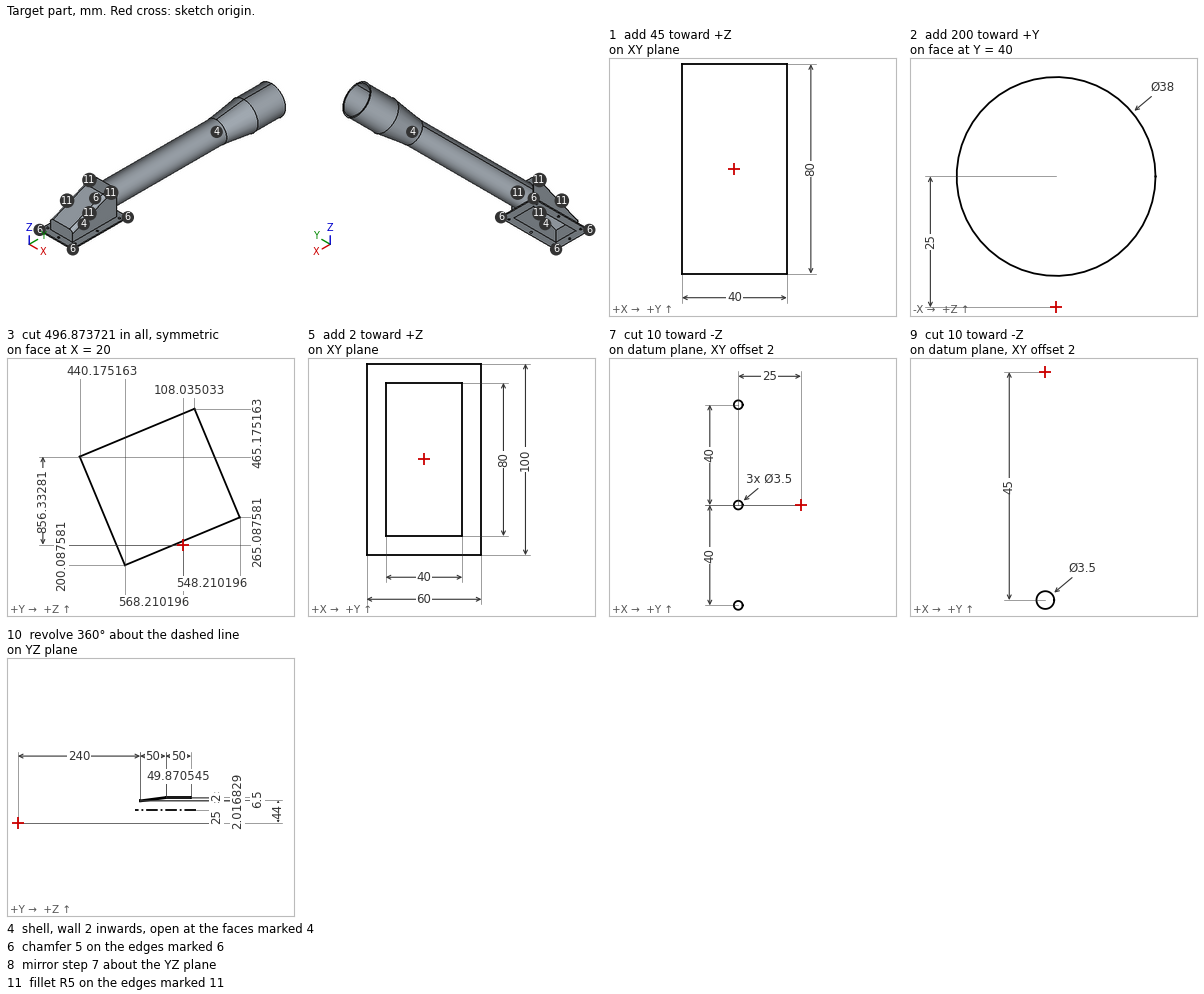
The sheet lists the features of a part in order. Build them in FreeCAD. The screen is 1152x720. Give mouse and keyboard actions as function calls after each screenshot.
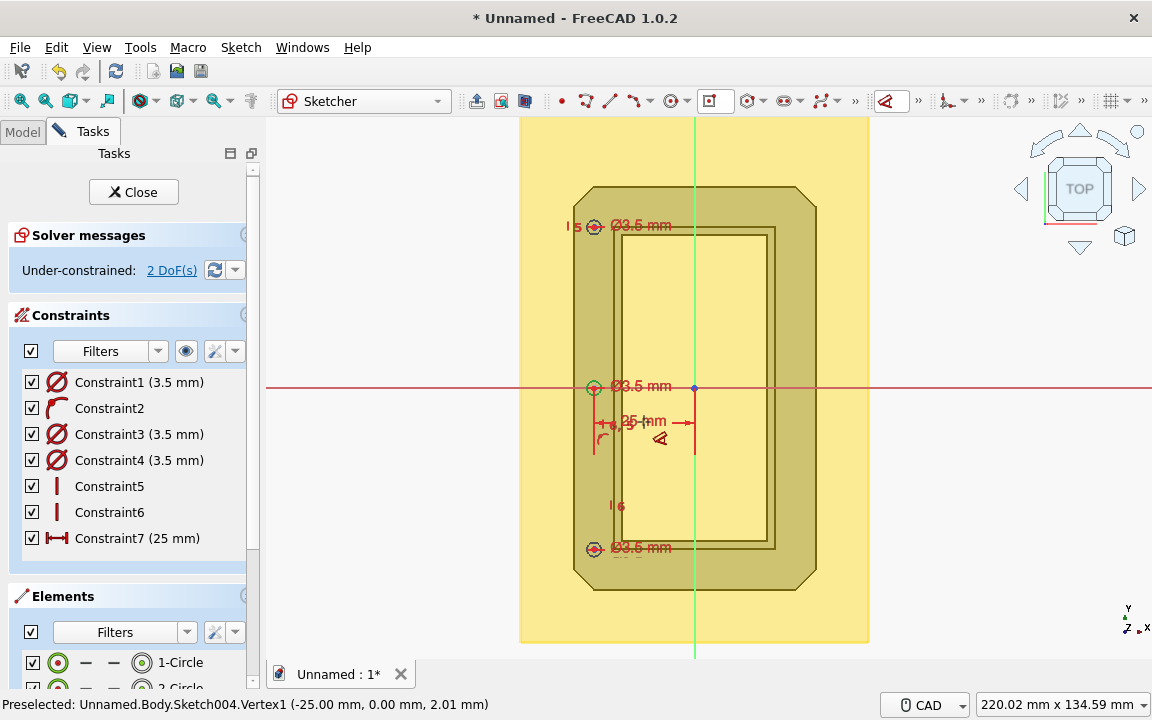
click(594, 227)
click(729, 308)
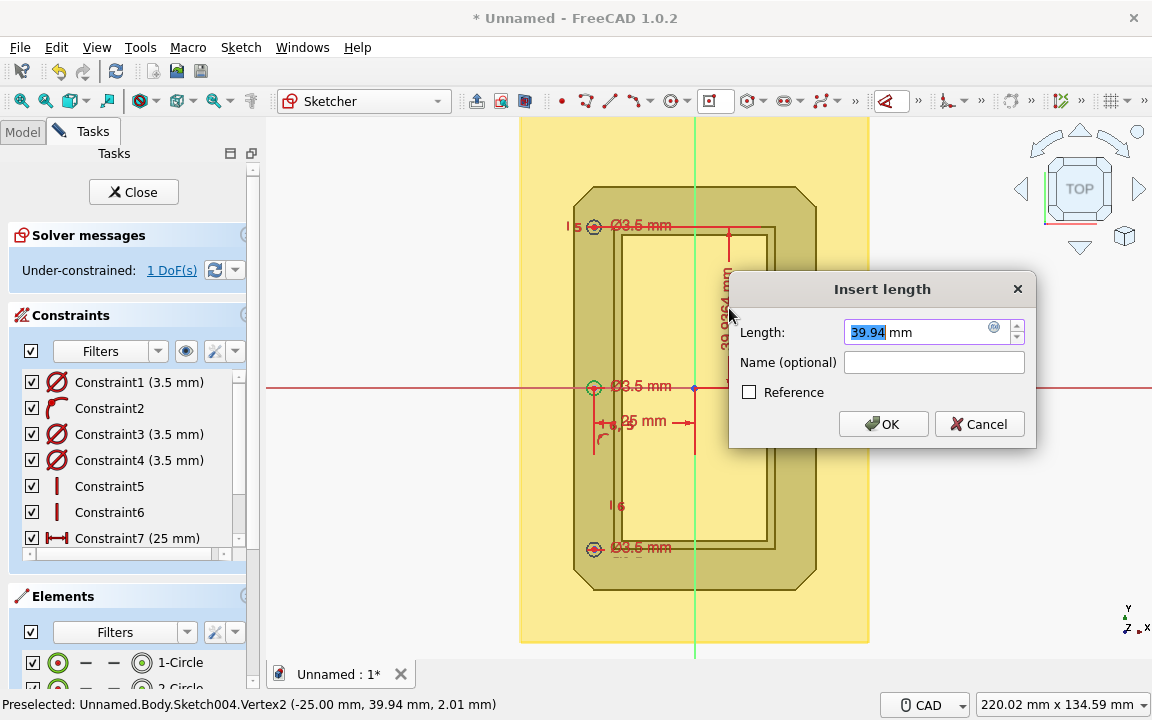
text(40)
key(Return)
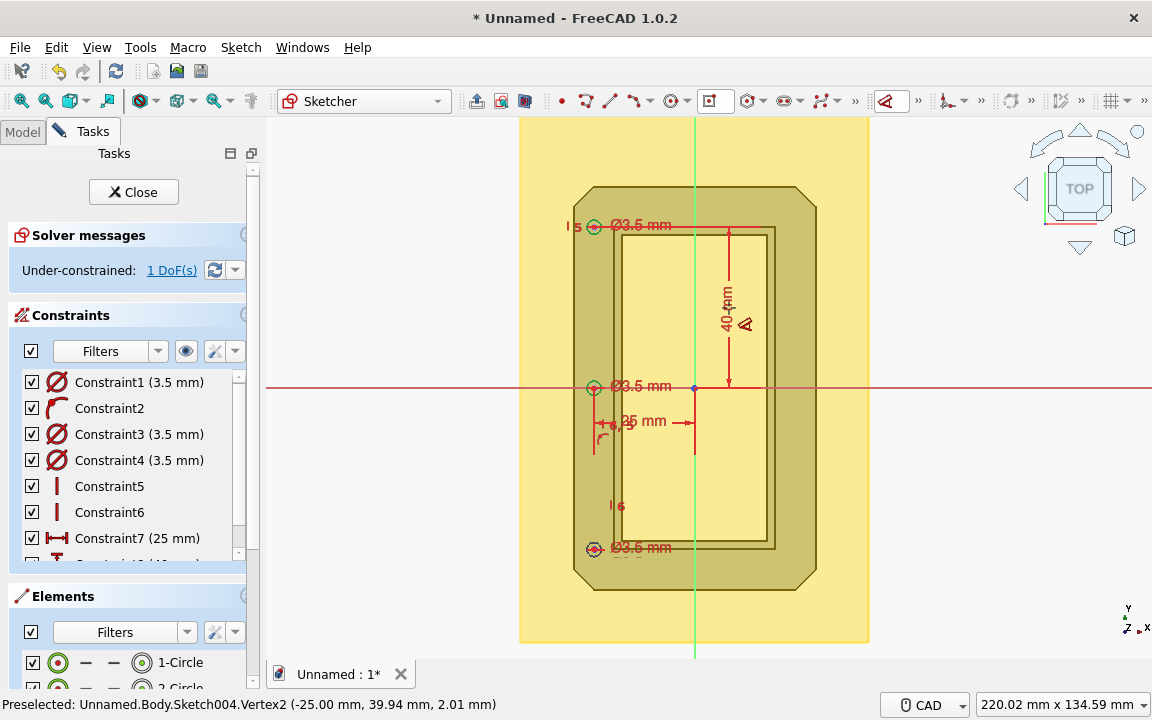
click(594, 550)
click(729, 469)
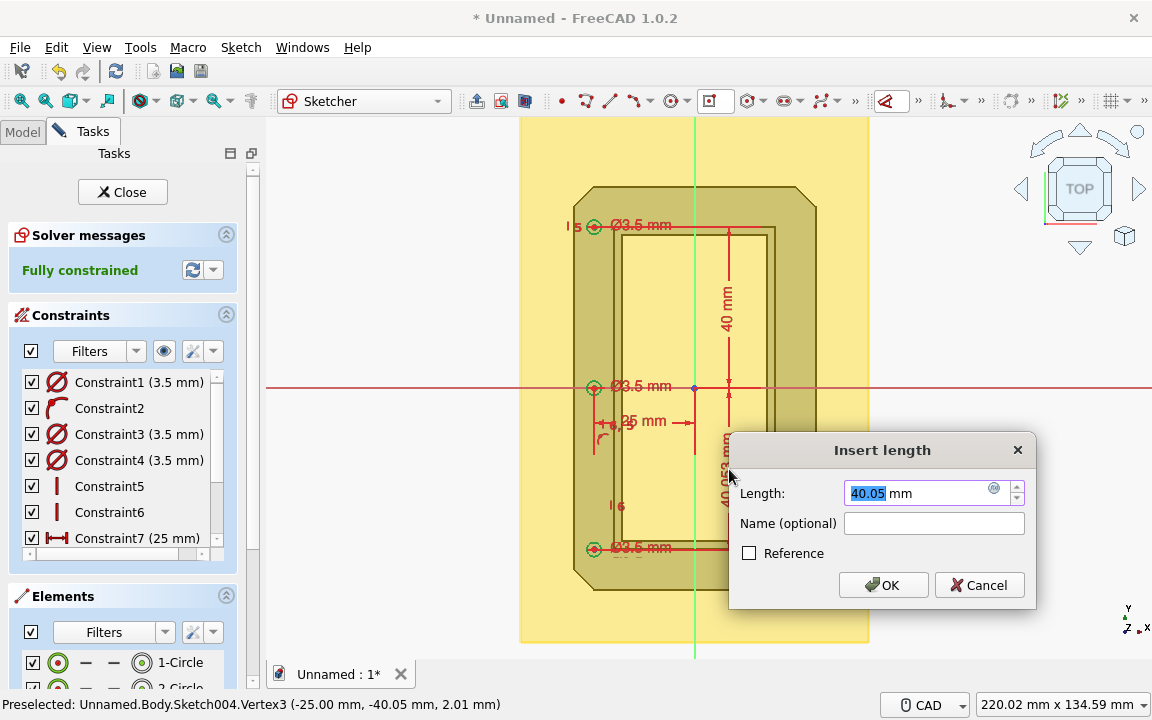
text(40)
key(Return)
key(Escape)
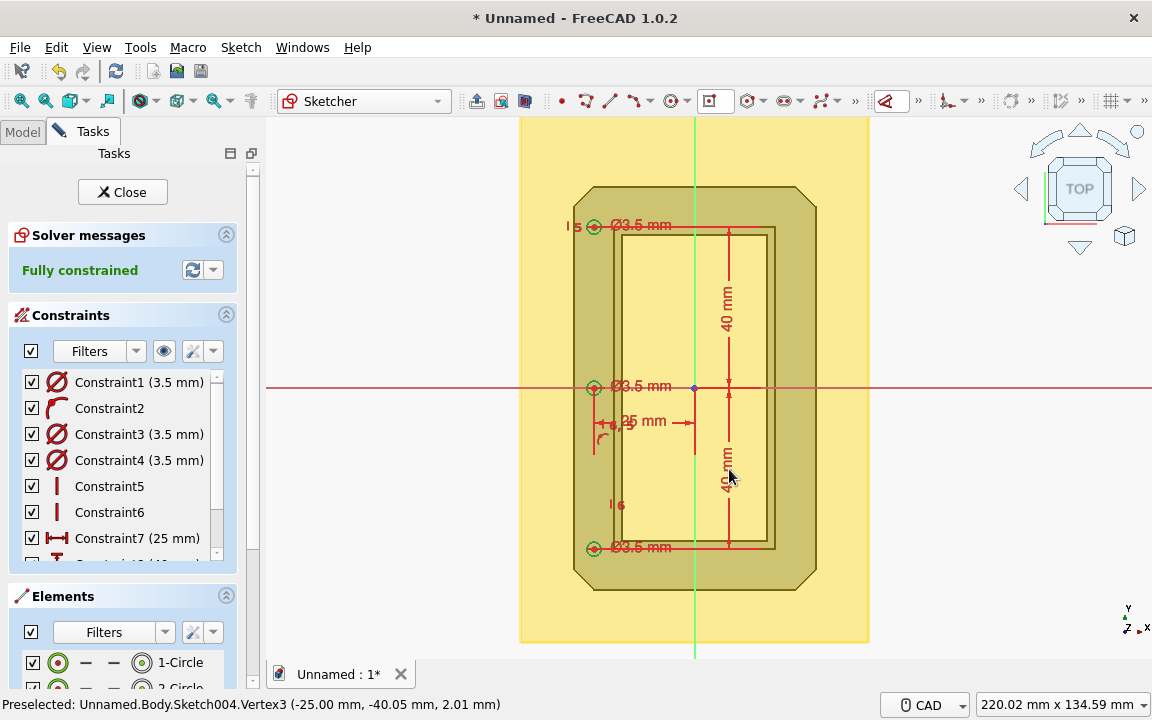
click(123, 192)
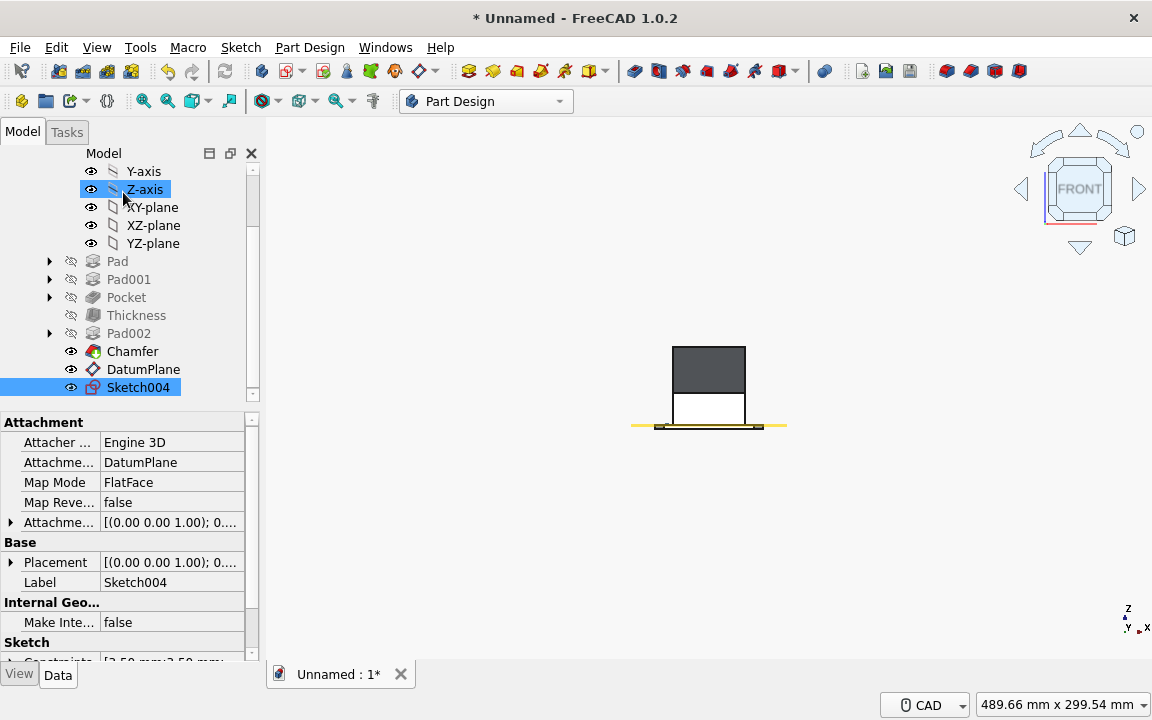
click(636, 72)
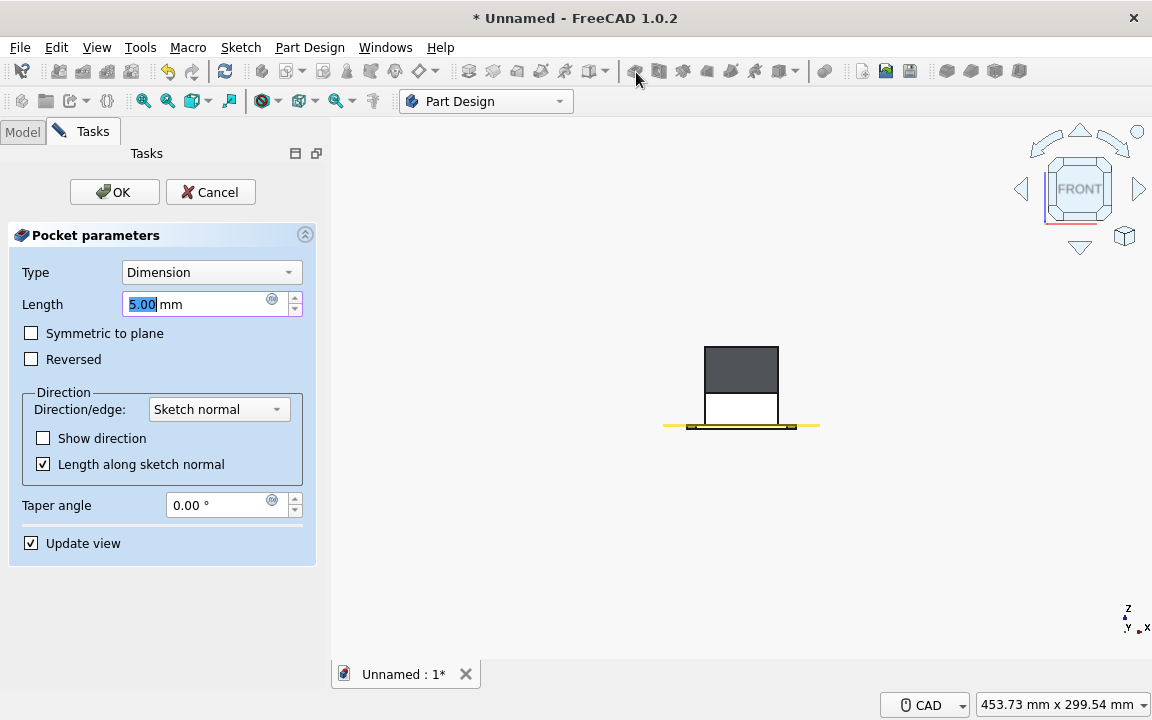
text(10)
key(Tab)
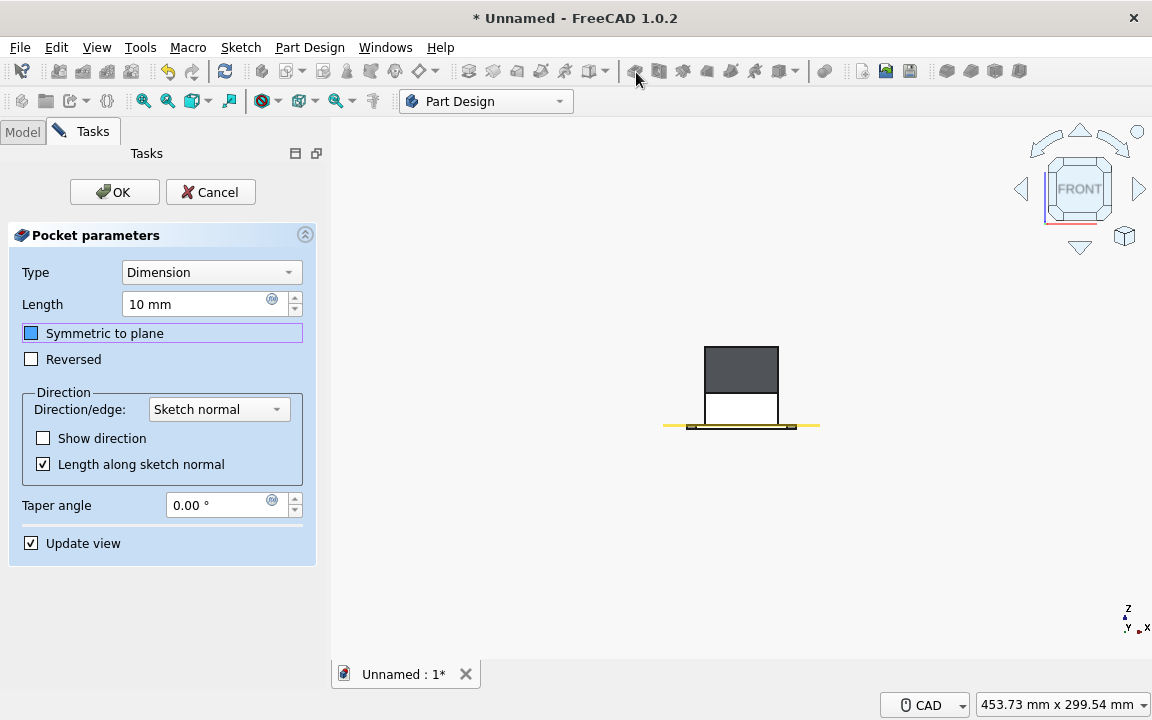
click(115, 192)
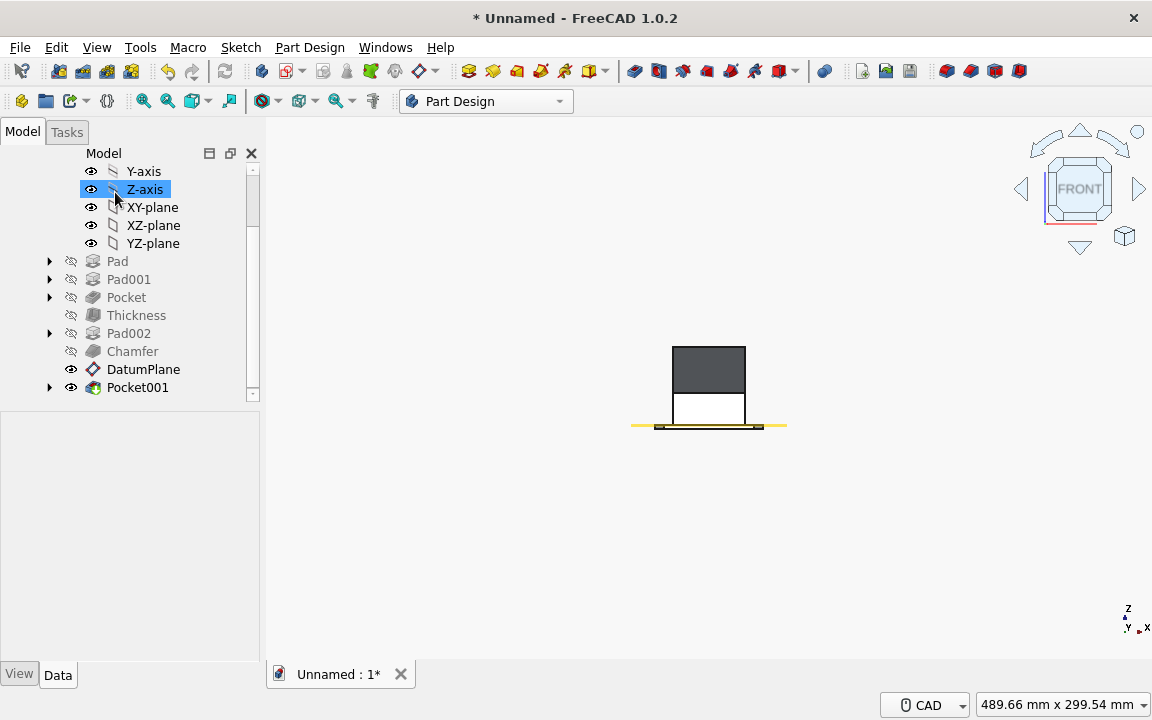
click(116, 369)
key(space)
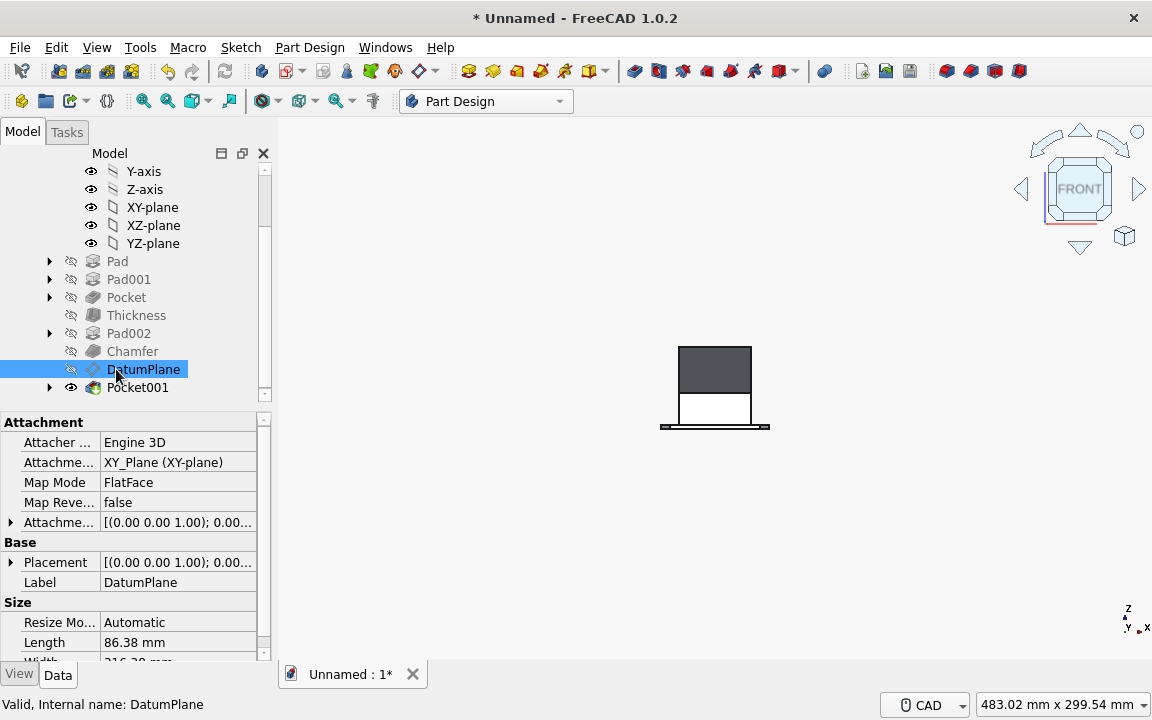
key(v)
key(f)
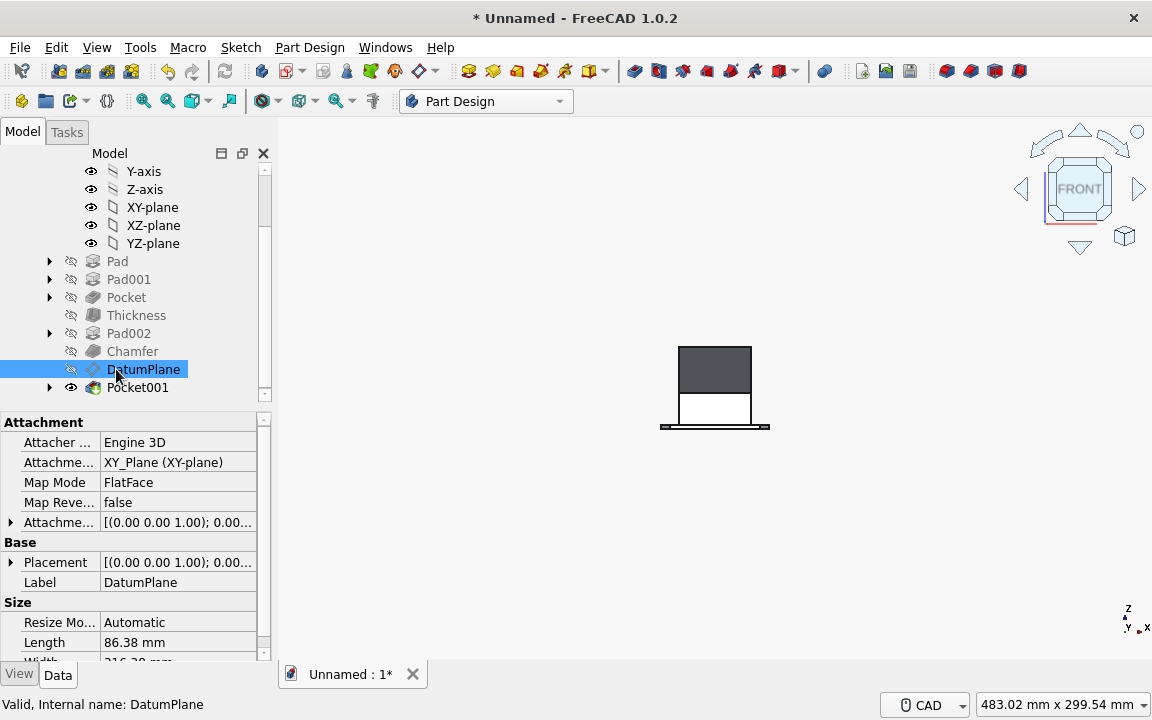
click(116, 387)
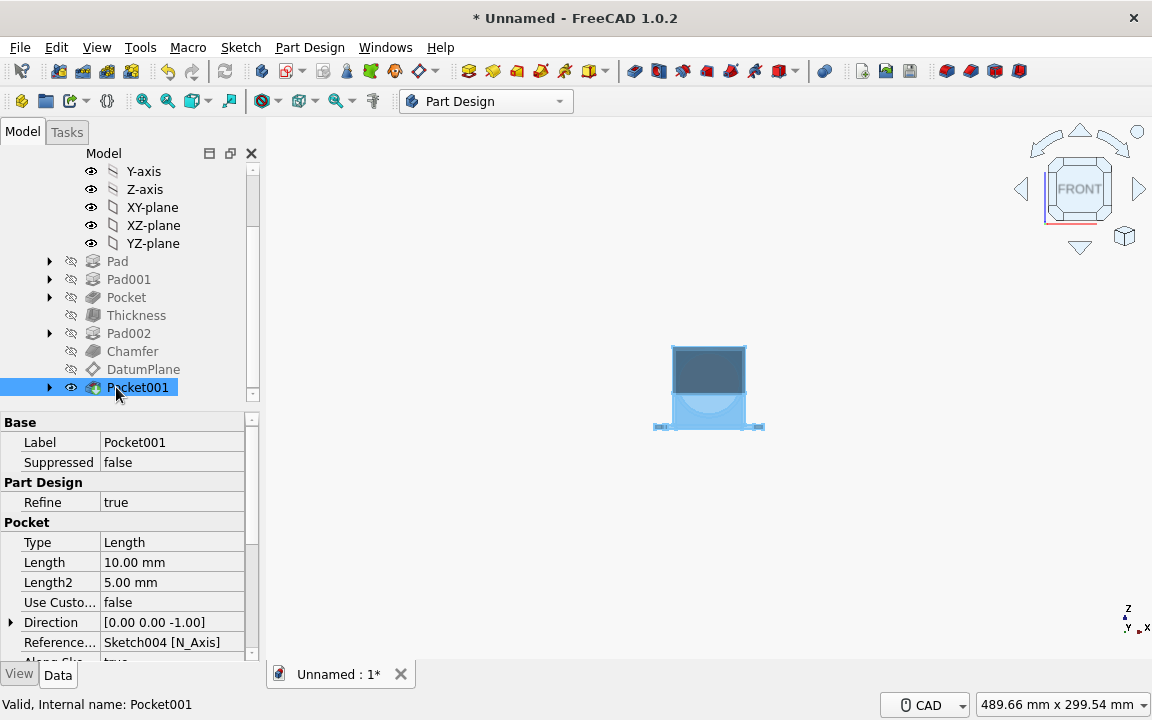
click(60, 72)